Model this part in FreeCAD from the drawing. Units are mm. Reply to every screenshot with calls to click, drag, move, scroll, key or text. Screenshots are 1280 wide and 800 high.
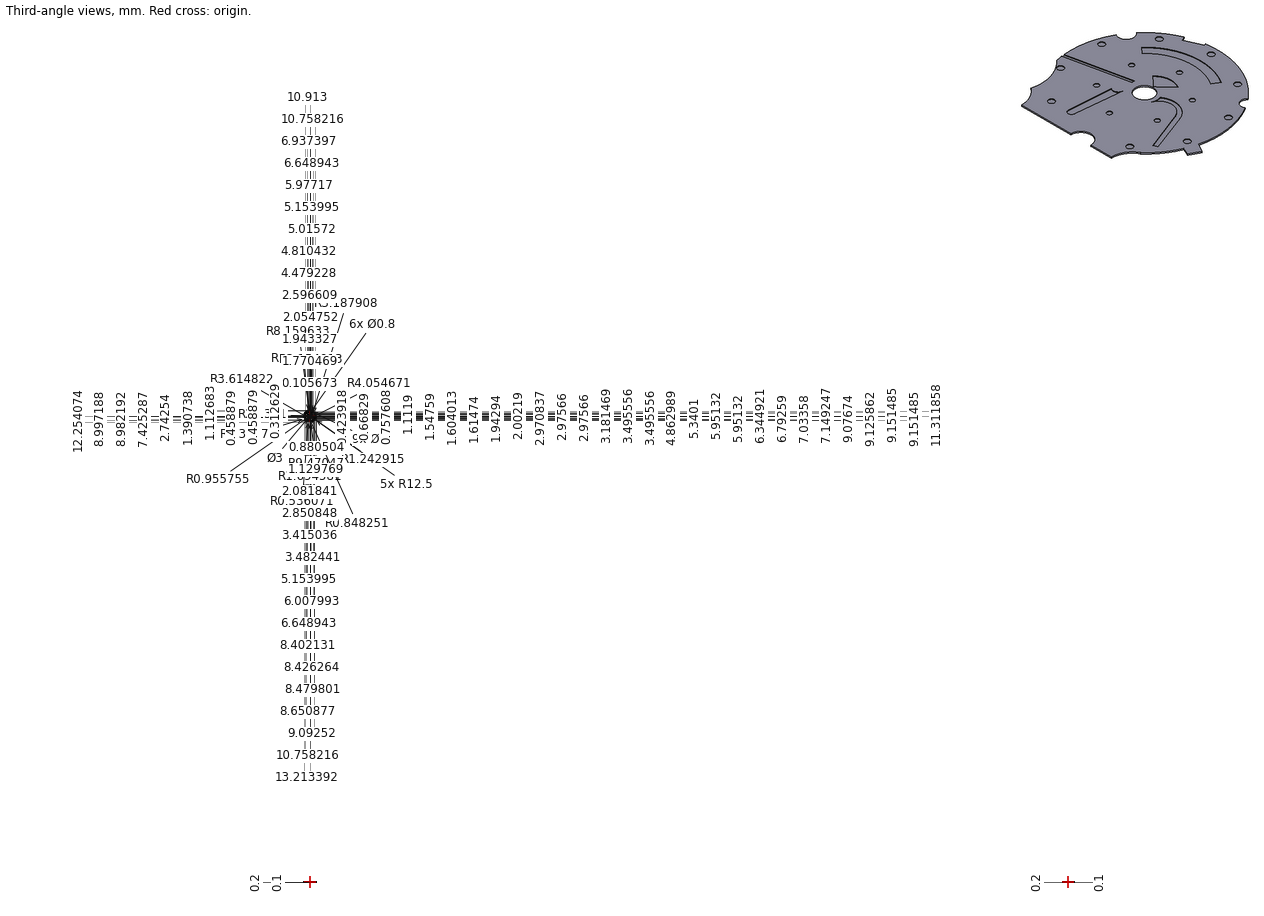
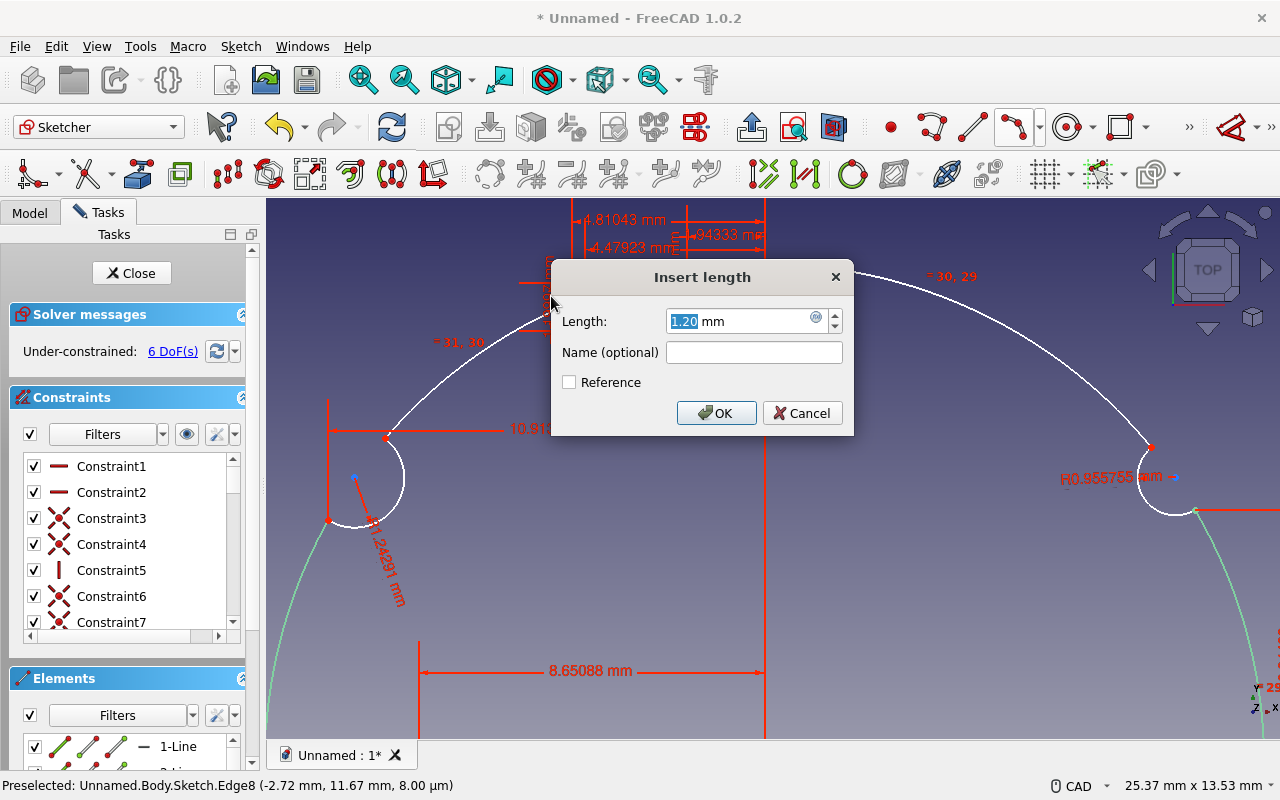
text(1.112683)
key(Return)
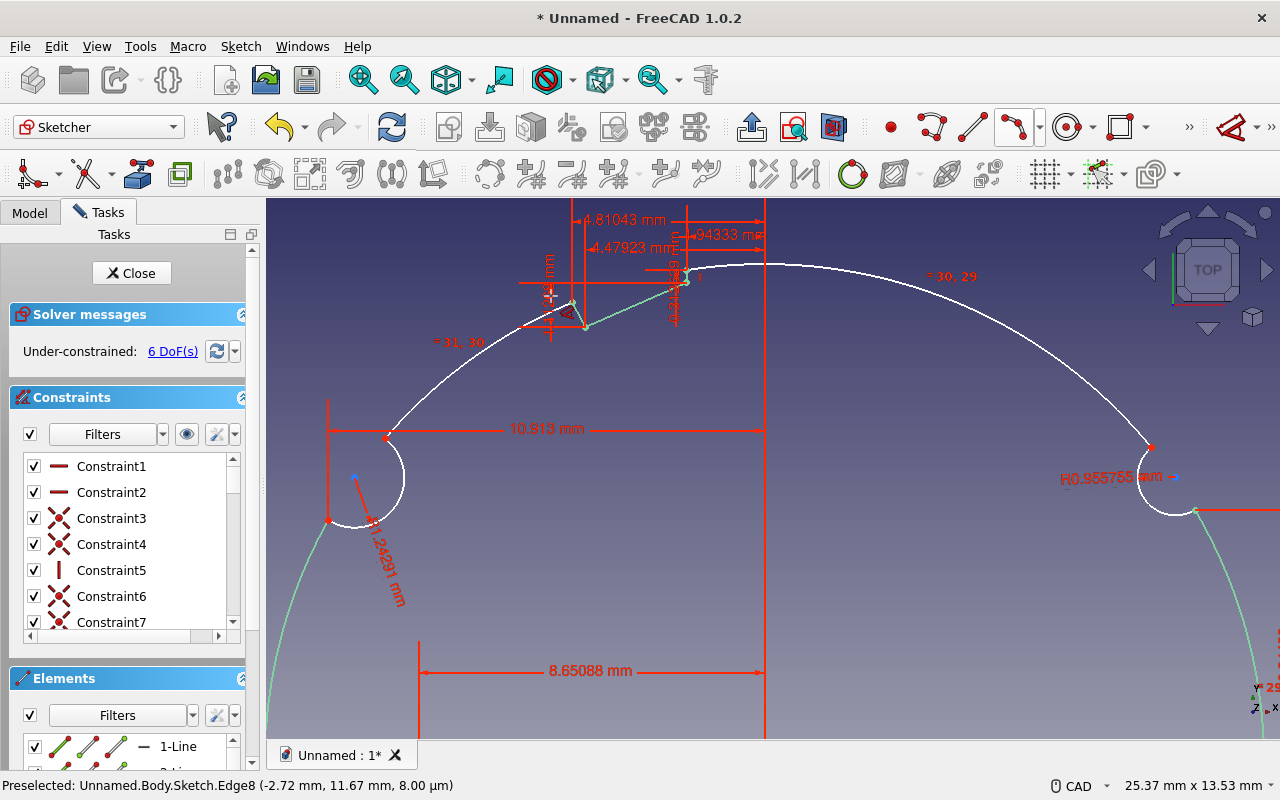
scroll(656, 298, down, 5)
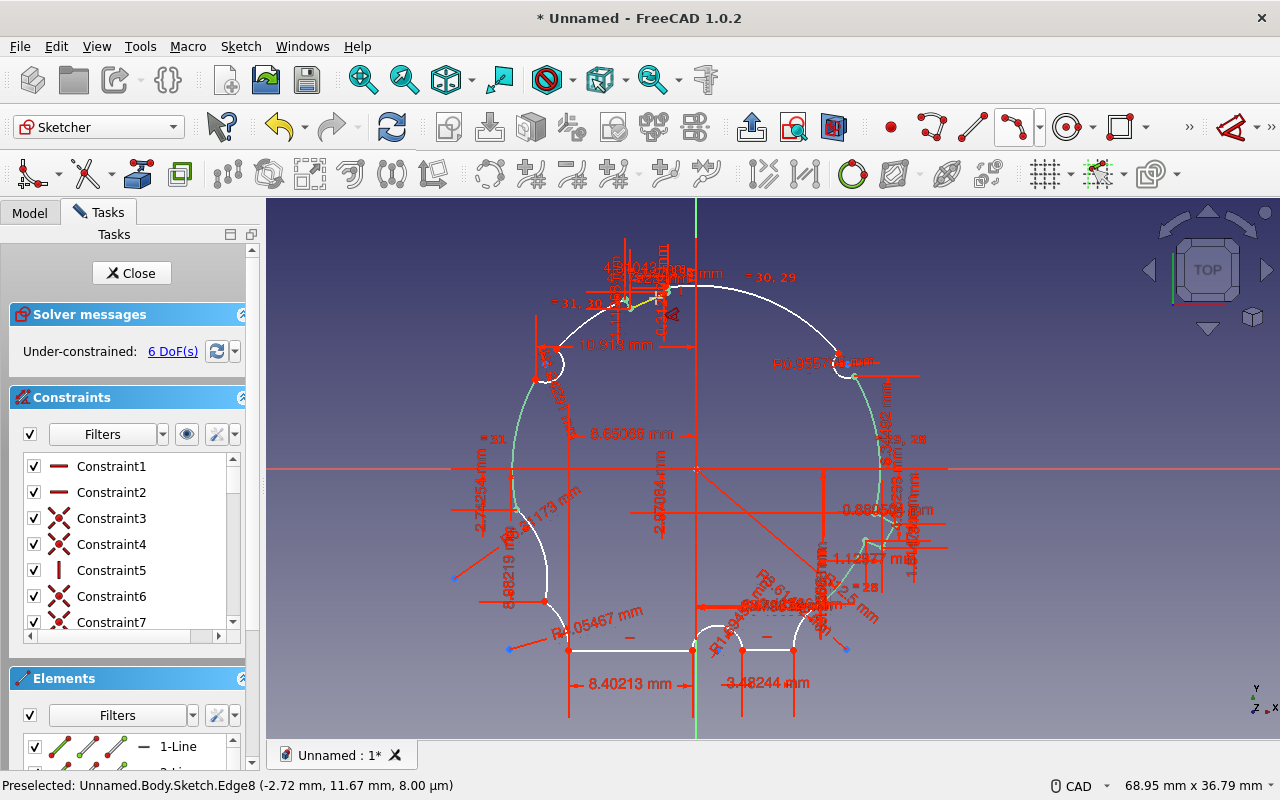
click(847, 364)
click(881, 392)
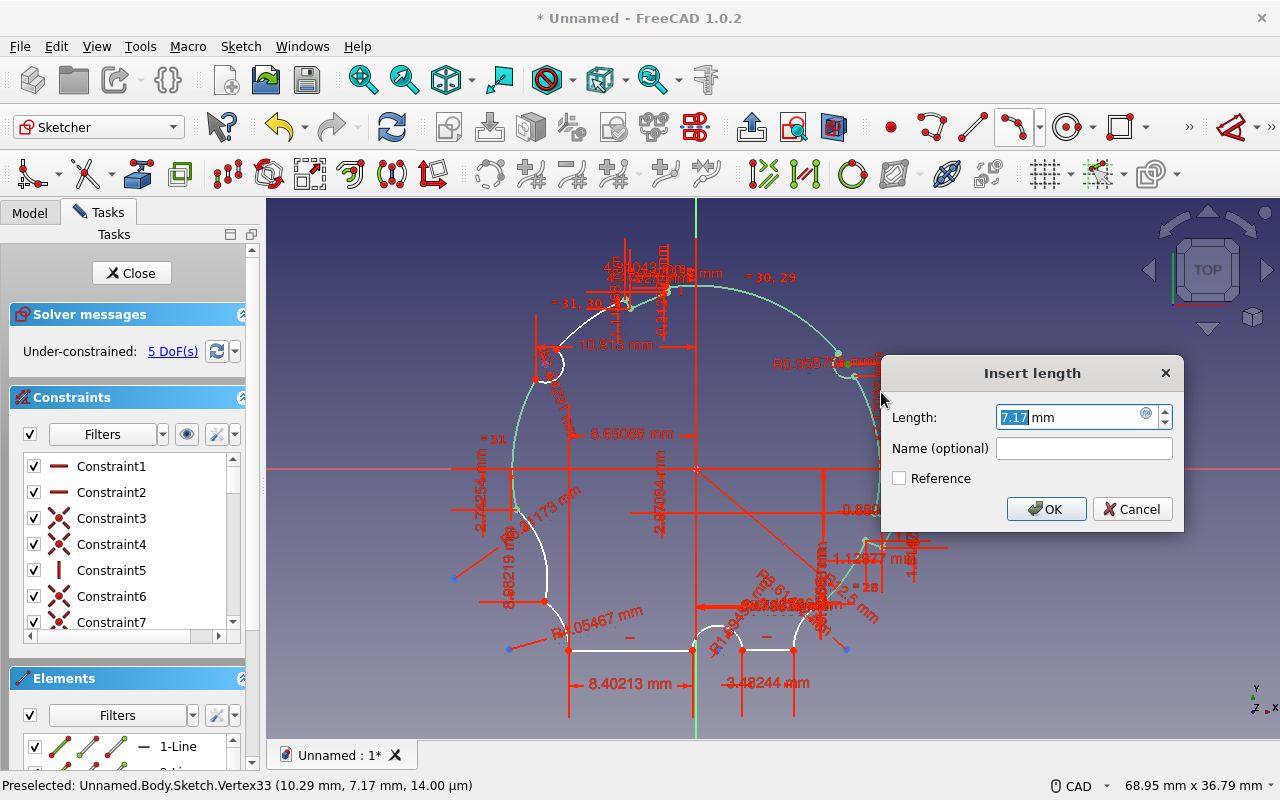
text(7.149247)
key(Return)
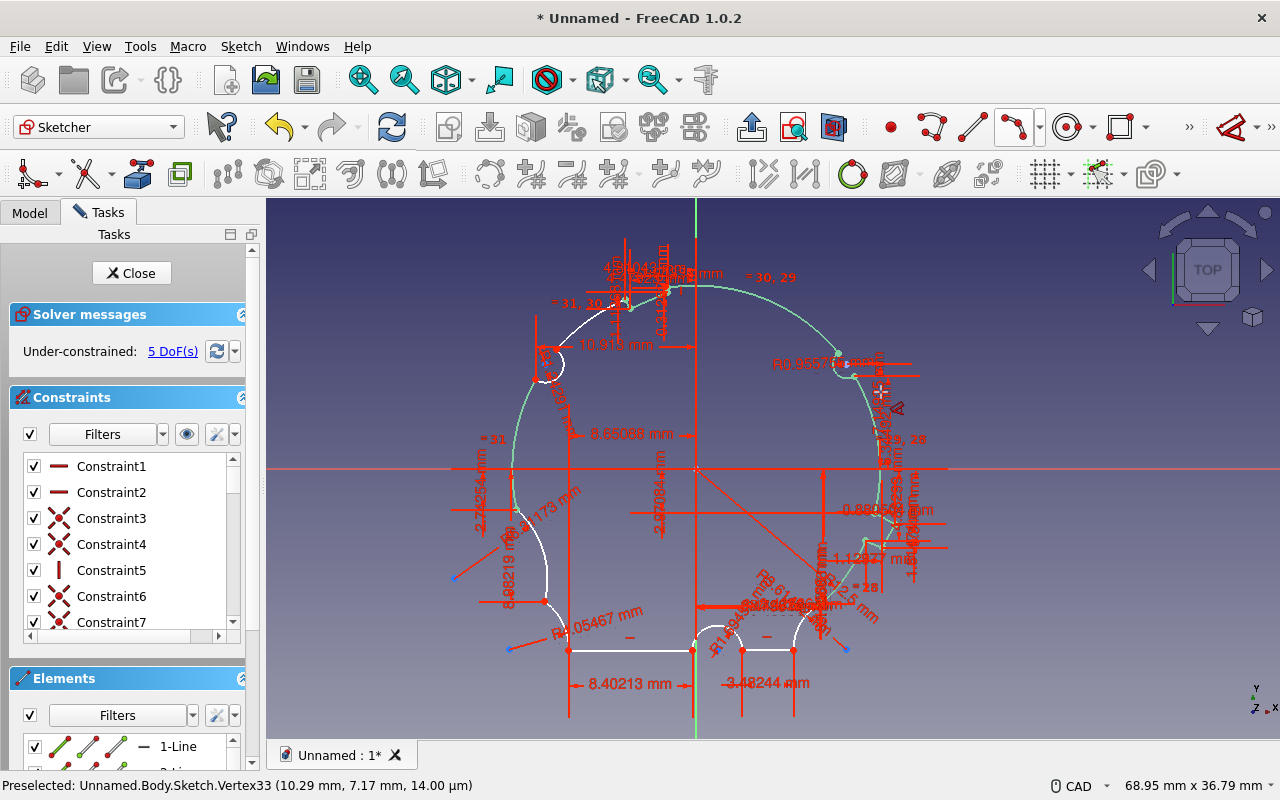
click(545, 364)
click(730, 417)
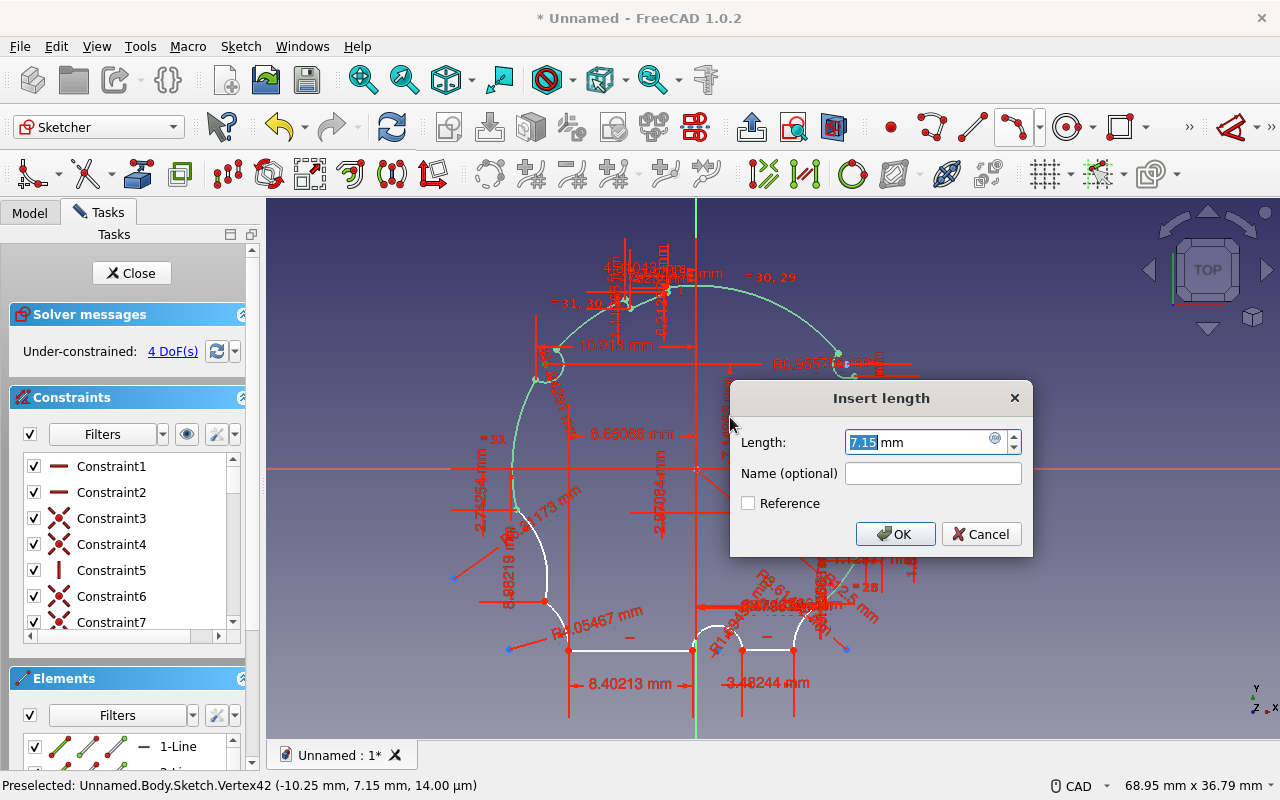
text(7.149247)
key(Return)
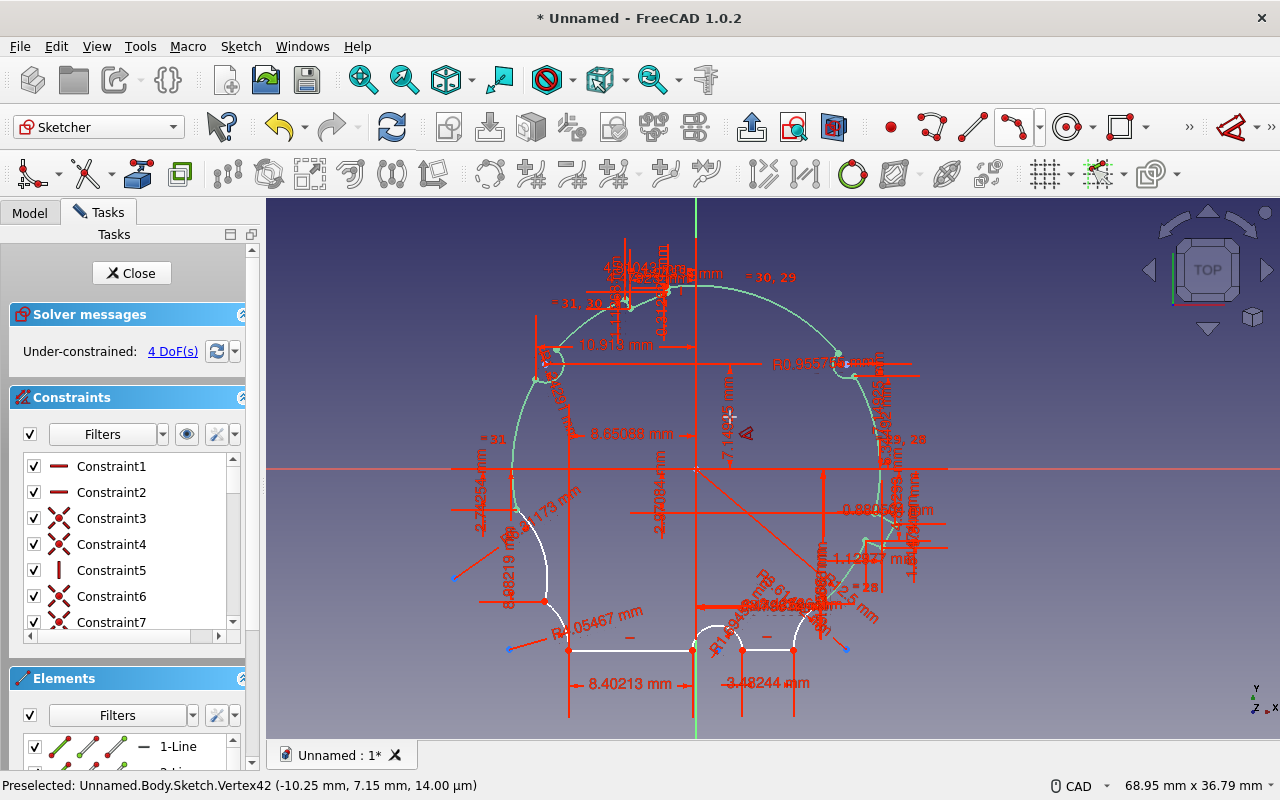
click(455, 579)
click(421, 524)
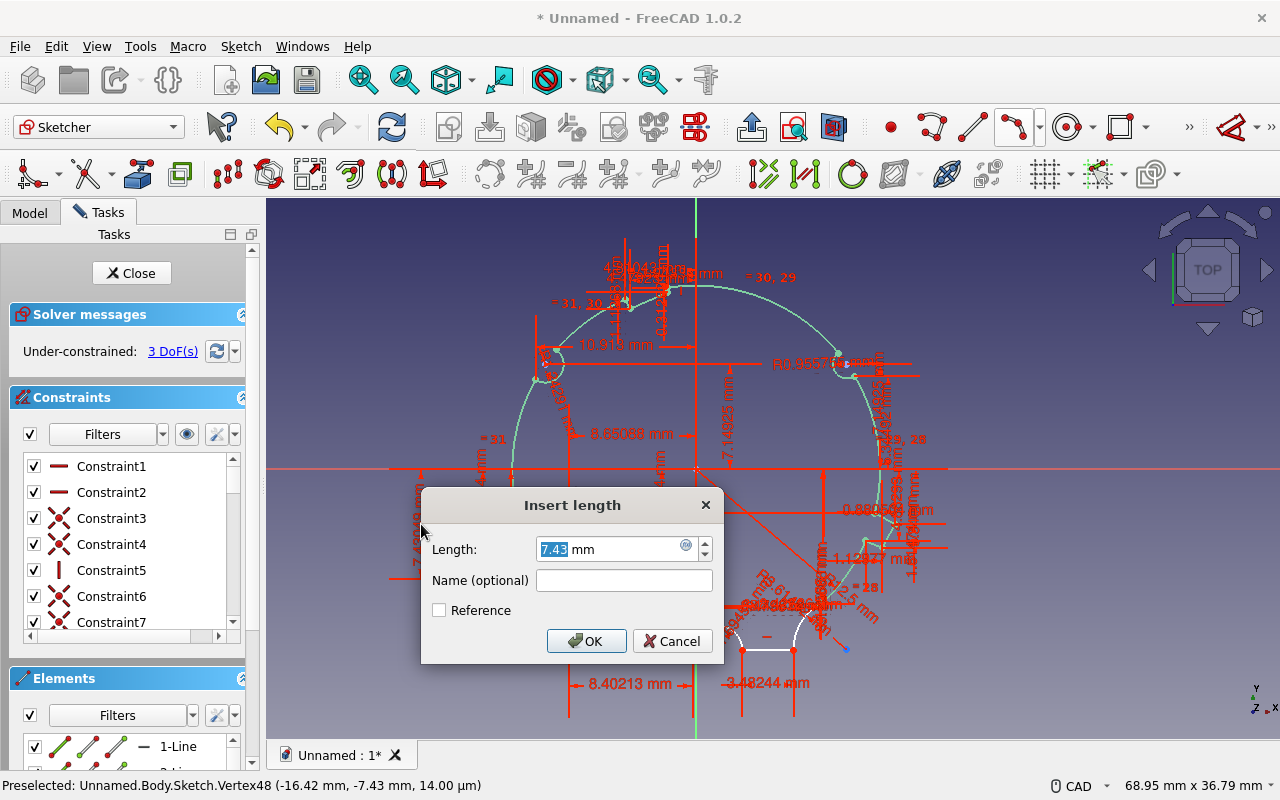
text(7.425287)
key(Return)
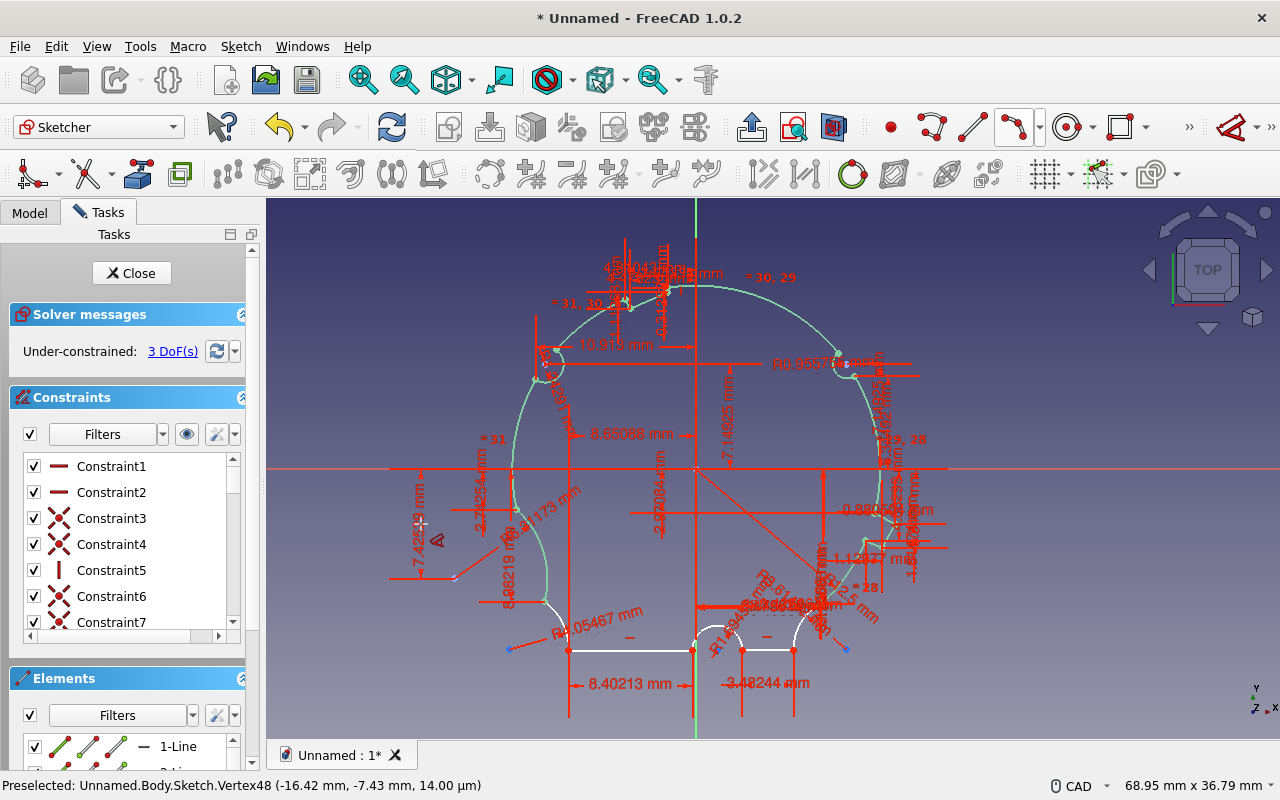
click(569, 651)
click(730, 560)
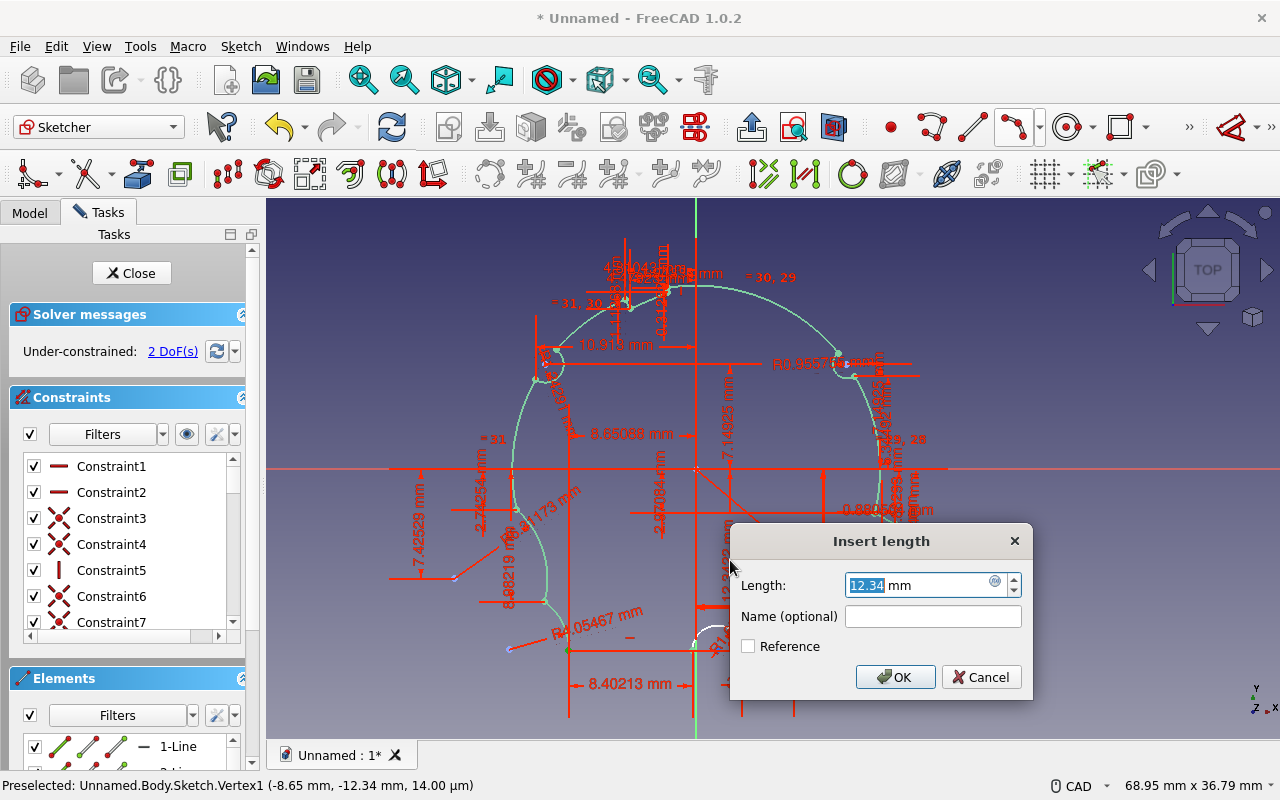
text(12.254074)
key(Return)